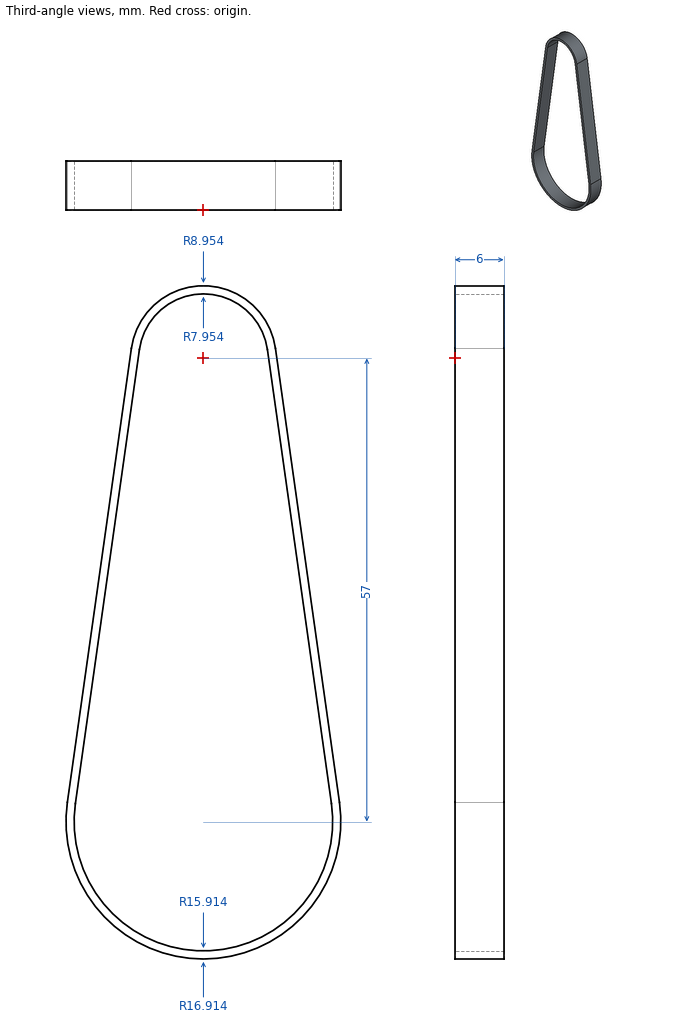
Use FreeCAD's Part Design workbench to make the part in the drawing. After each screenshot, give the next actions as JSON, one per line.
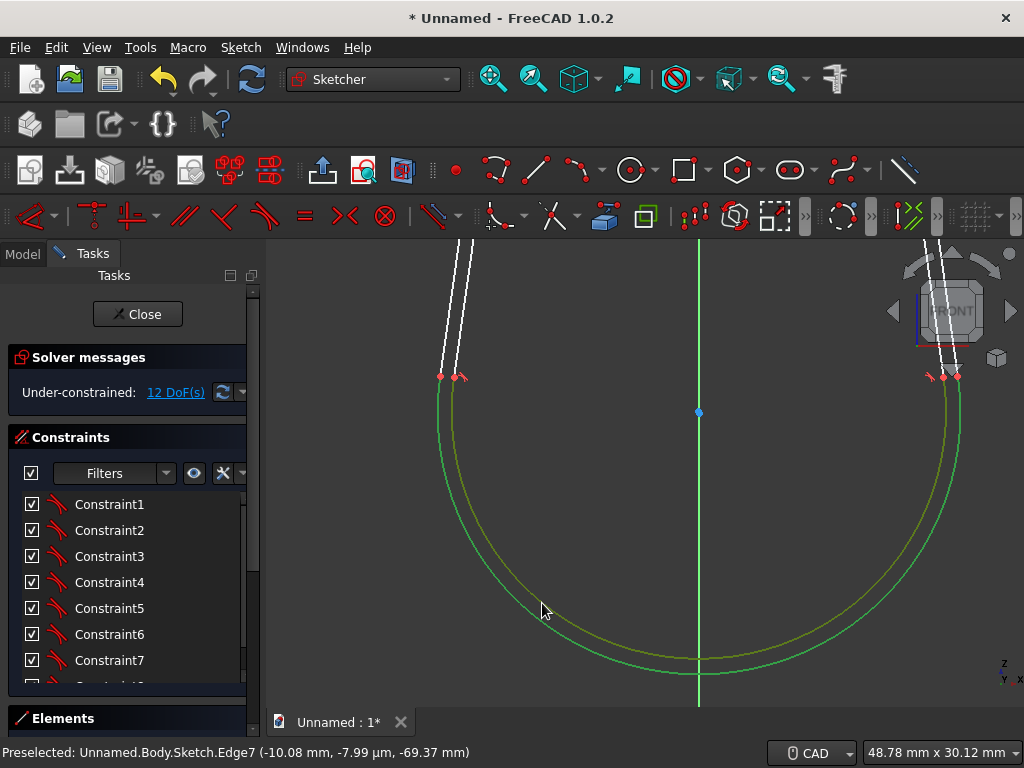
{"action": "left_click", "coordinate": [92, 216]}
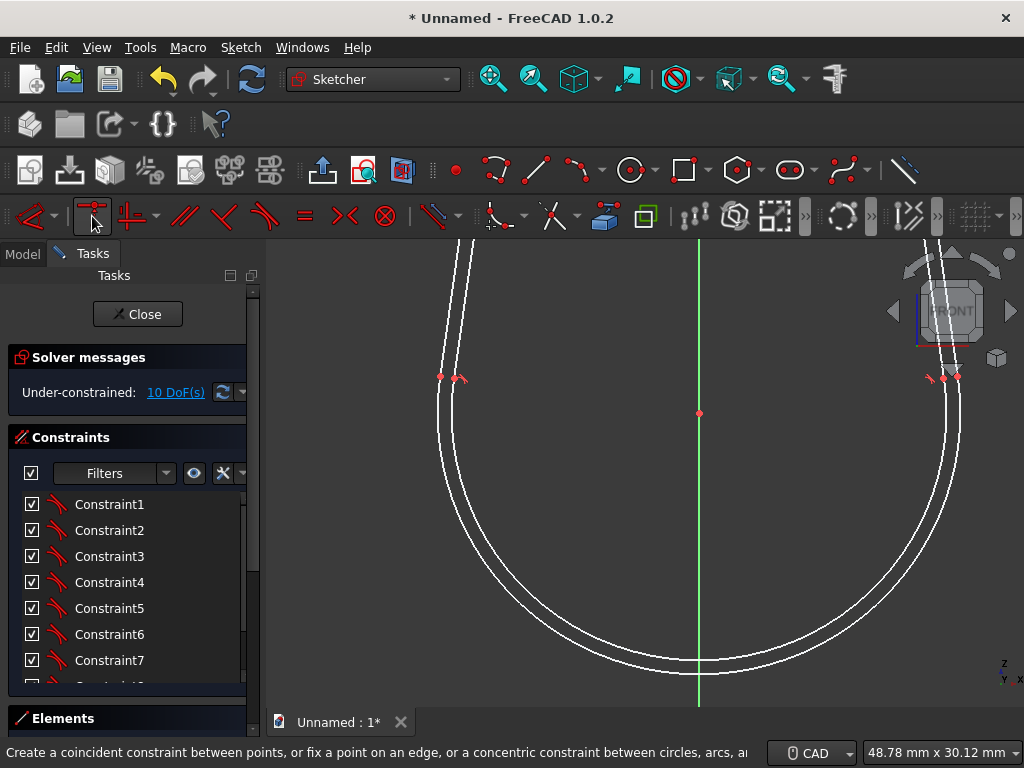
{"action": "scroll", "coordinate": [536, 618], "scroll_direction": "down", "scroll_amount": 7}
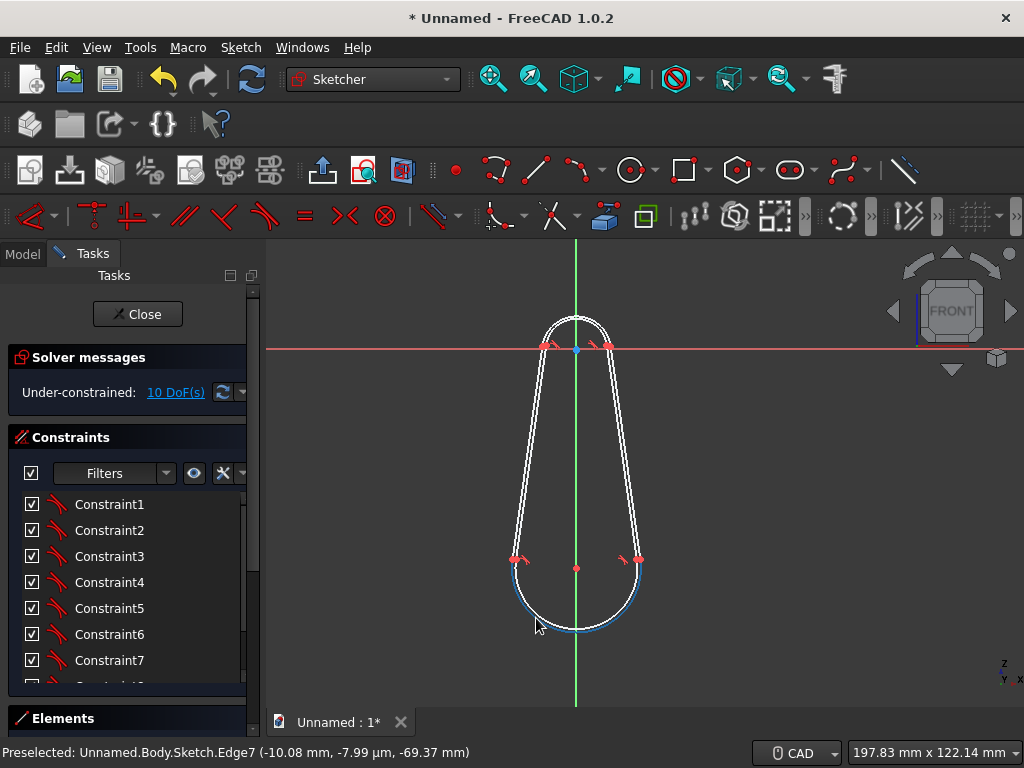
{"action": "scroll", "coordinate": [595, 322], "scroll_direction": "up", "scroll_amount": 9}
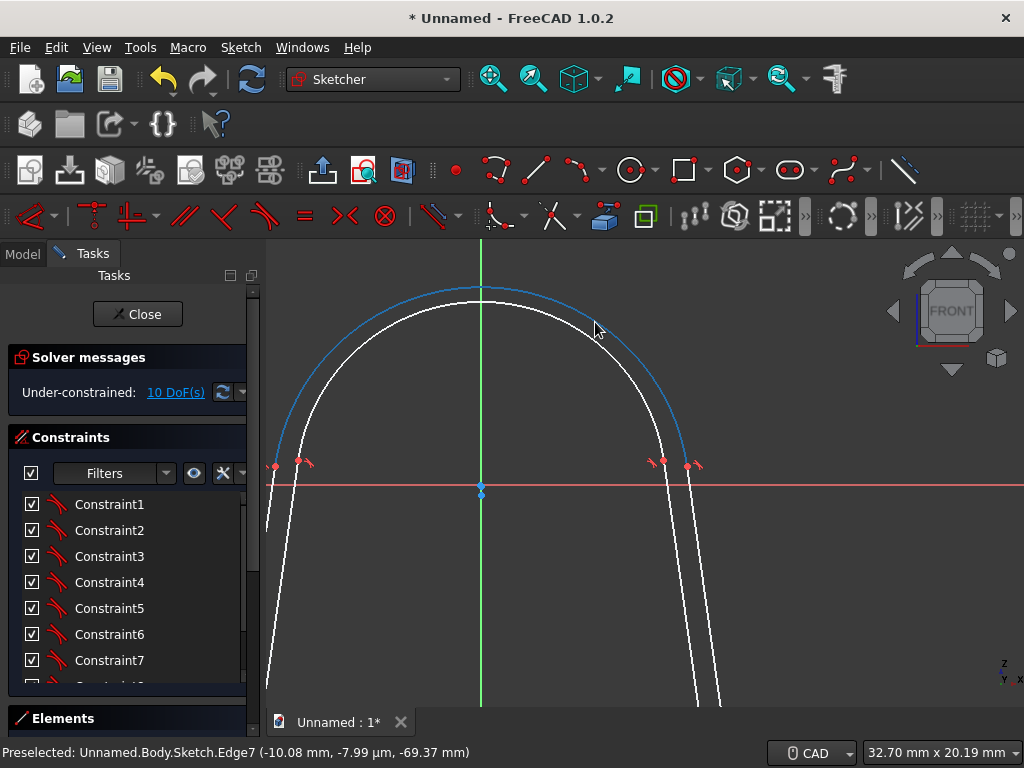
{"action": "left_click", "coordinate": [594, 320]}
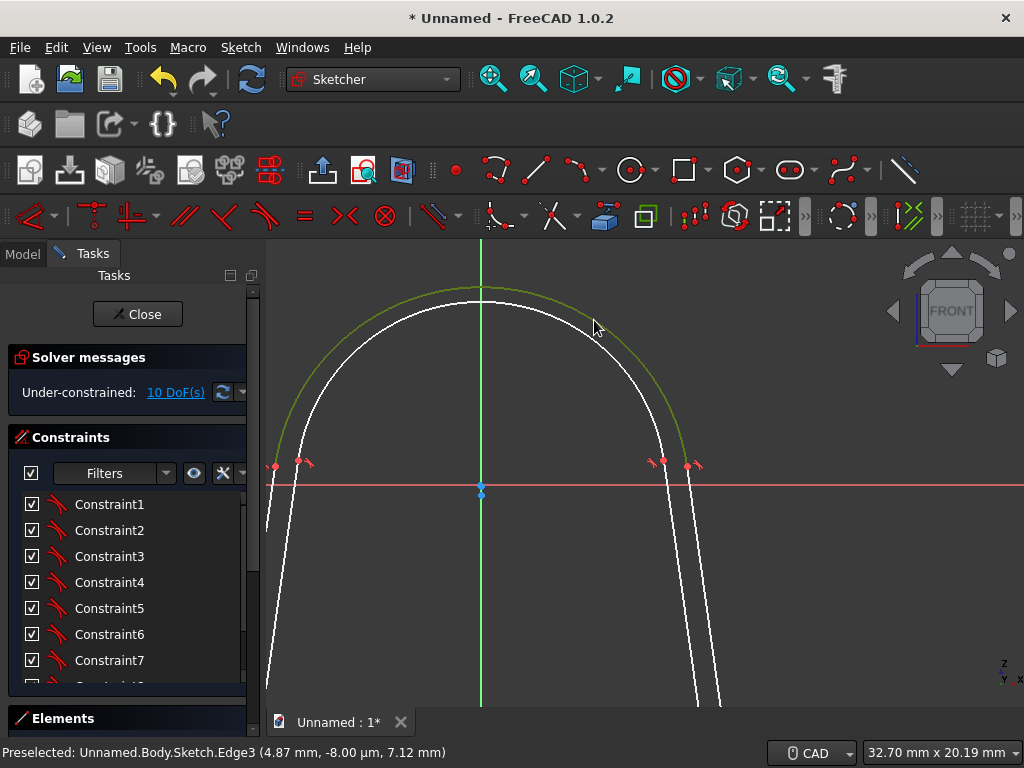
{"action": "left_click", "coordinate": [581, 331]}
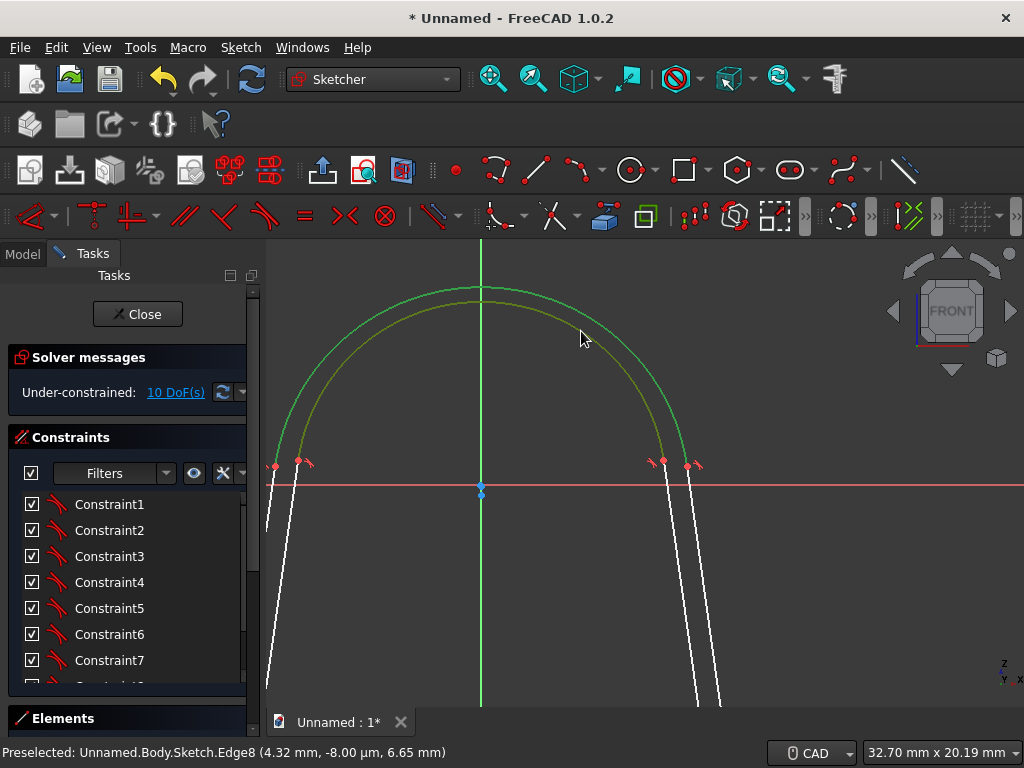
{"action": "left_click", "coordinate": [92, 216]}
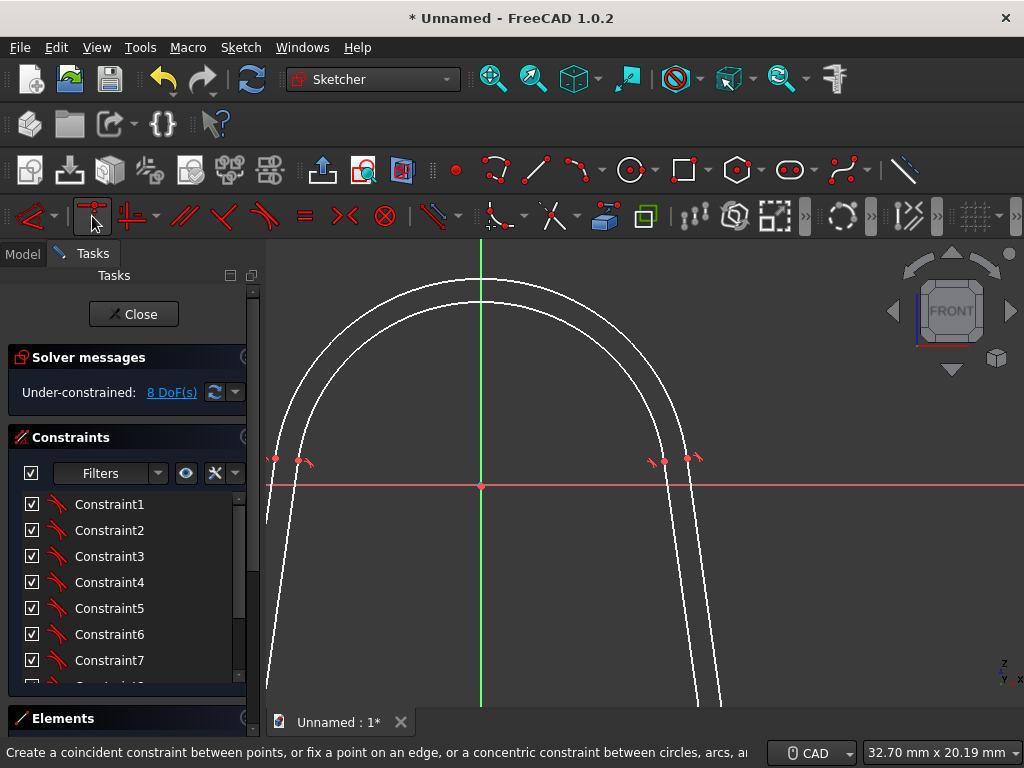
{"action": "scroll", "coordinate": [595, 321], "scroll_direction": "down", "scroll_amount": 9}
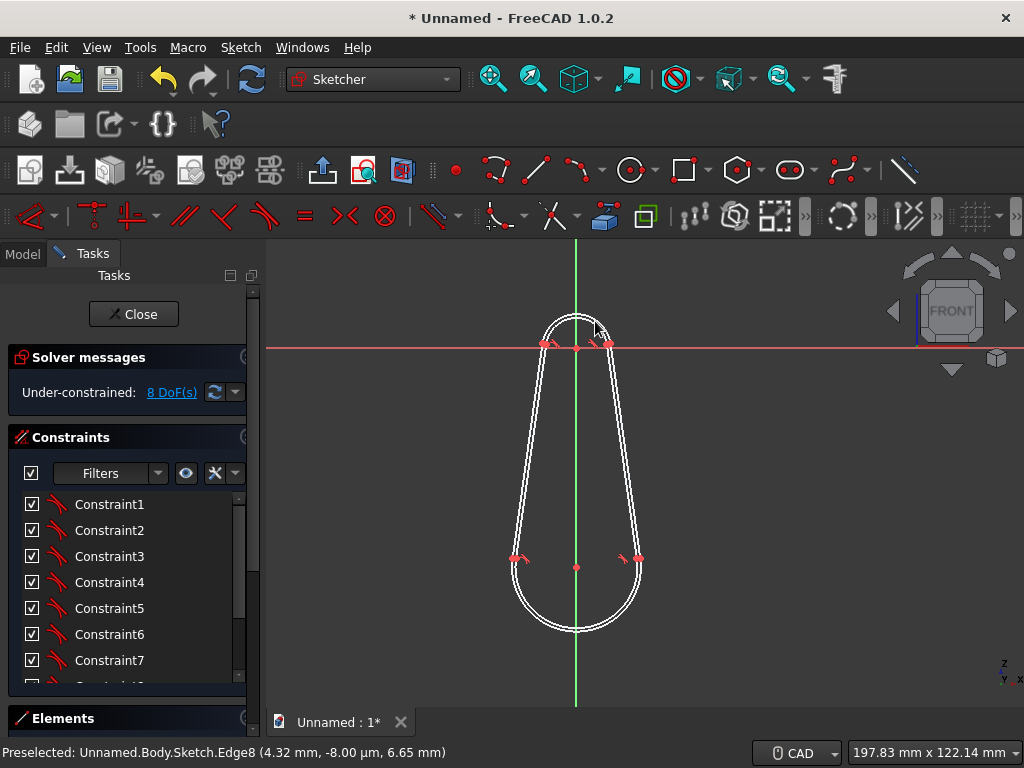
{"action": "scroll", "coordinate": [577, 348], "scroll_direction": "up", "scroll_amount": 2}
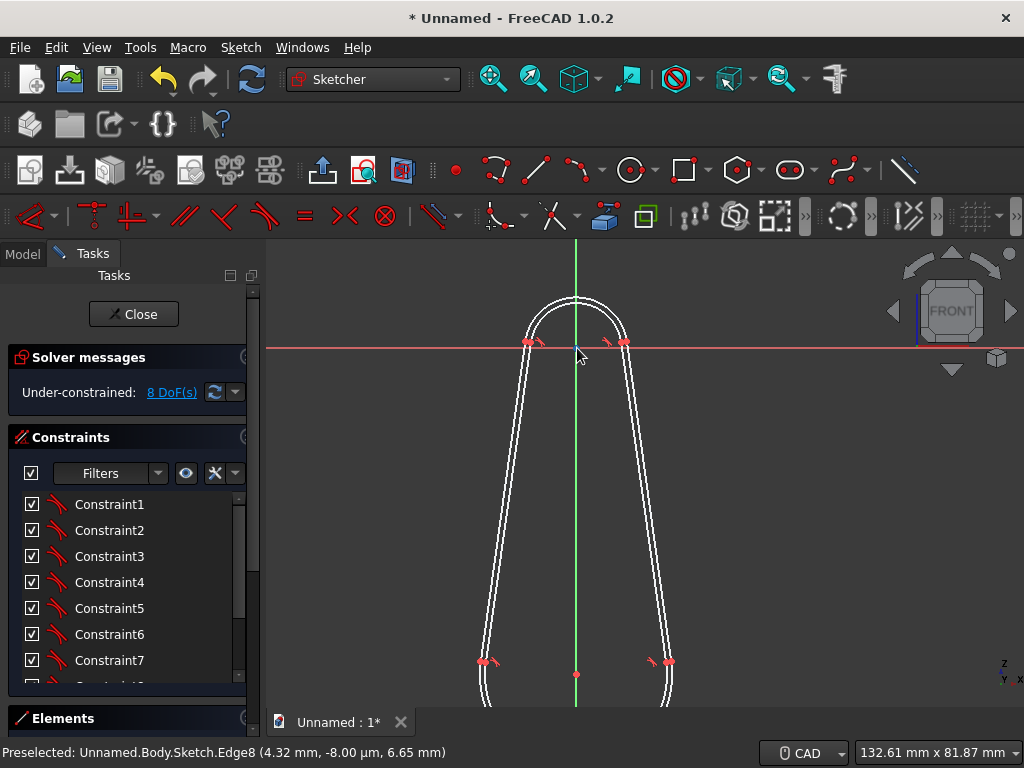
{"action": "left_click_drag", "start_coordinate": [566, 338], "coordinate": [586, 359]}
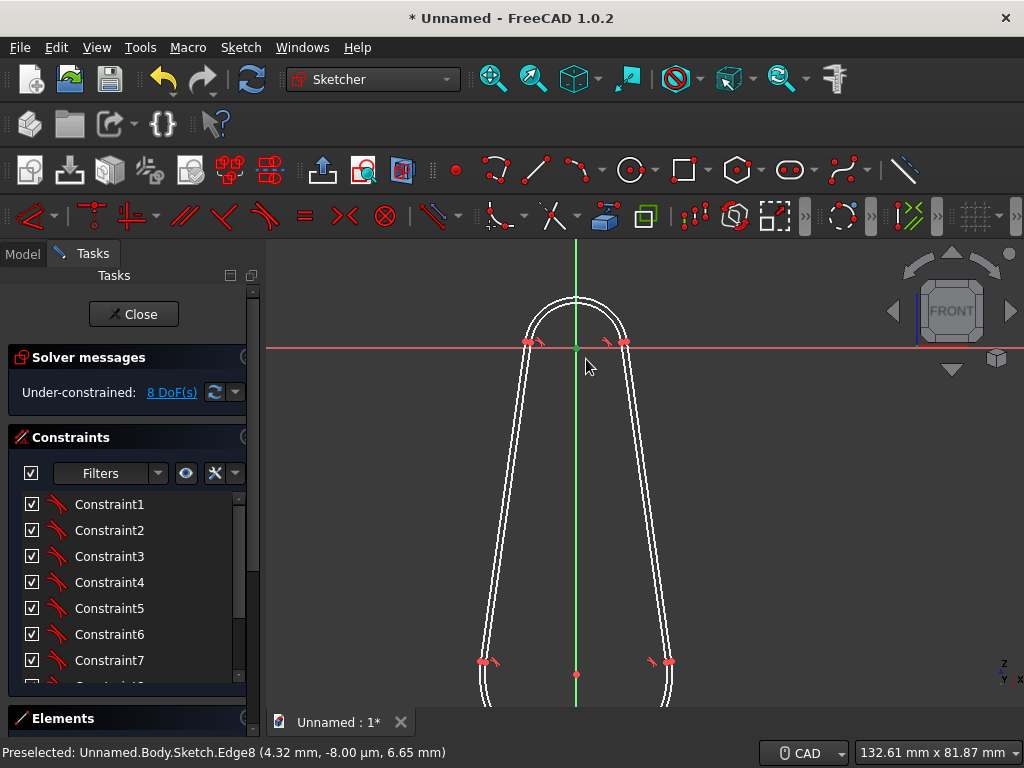
{"action": "left_click", "coordinate": [92, 216]}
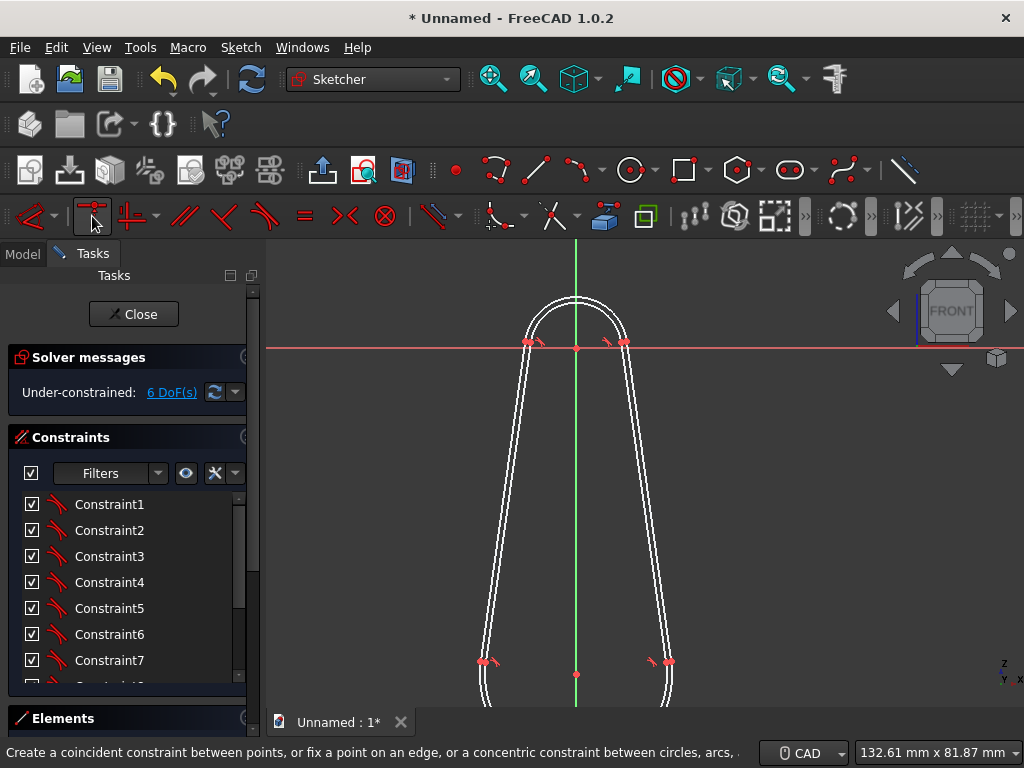
{"action": "left_click", "coordinate": [576, 675]}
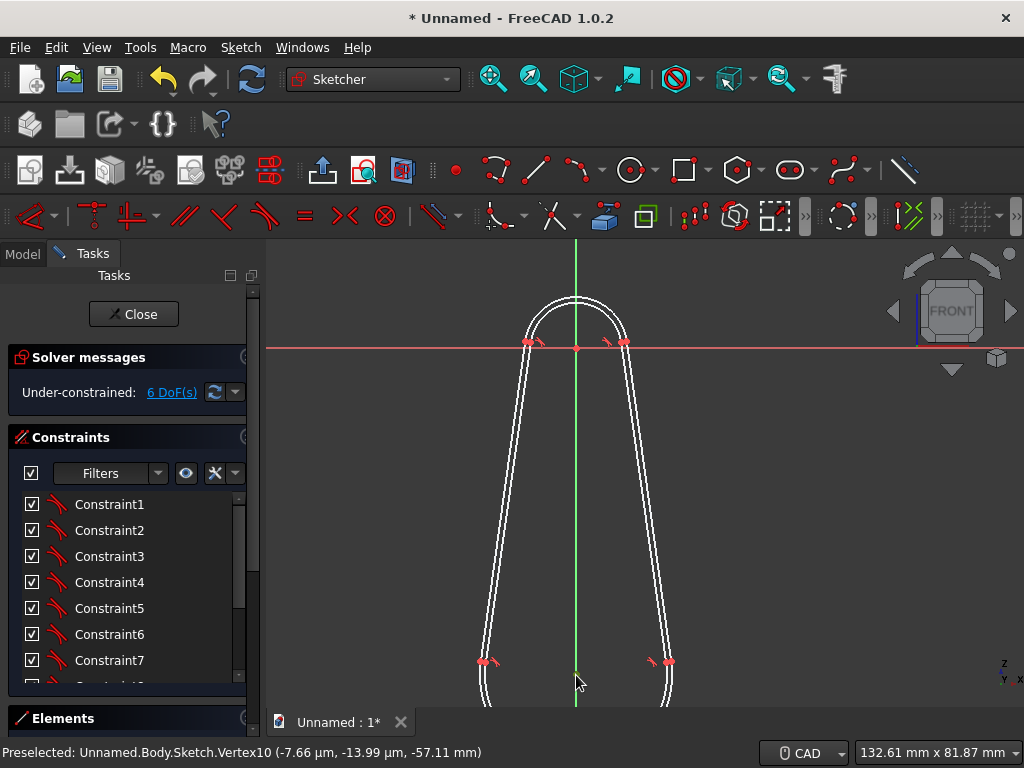
{"action": "left_click", "coordinate": [576, 650]}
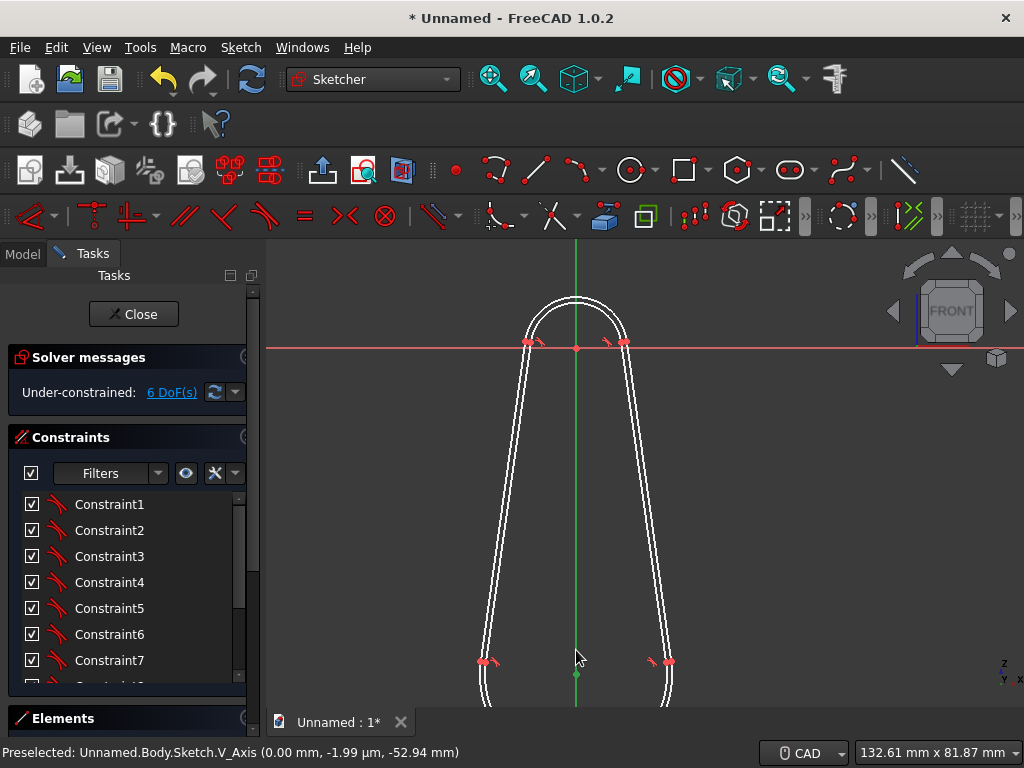
{"action": "left_click", "coordinate": [92, 216]}